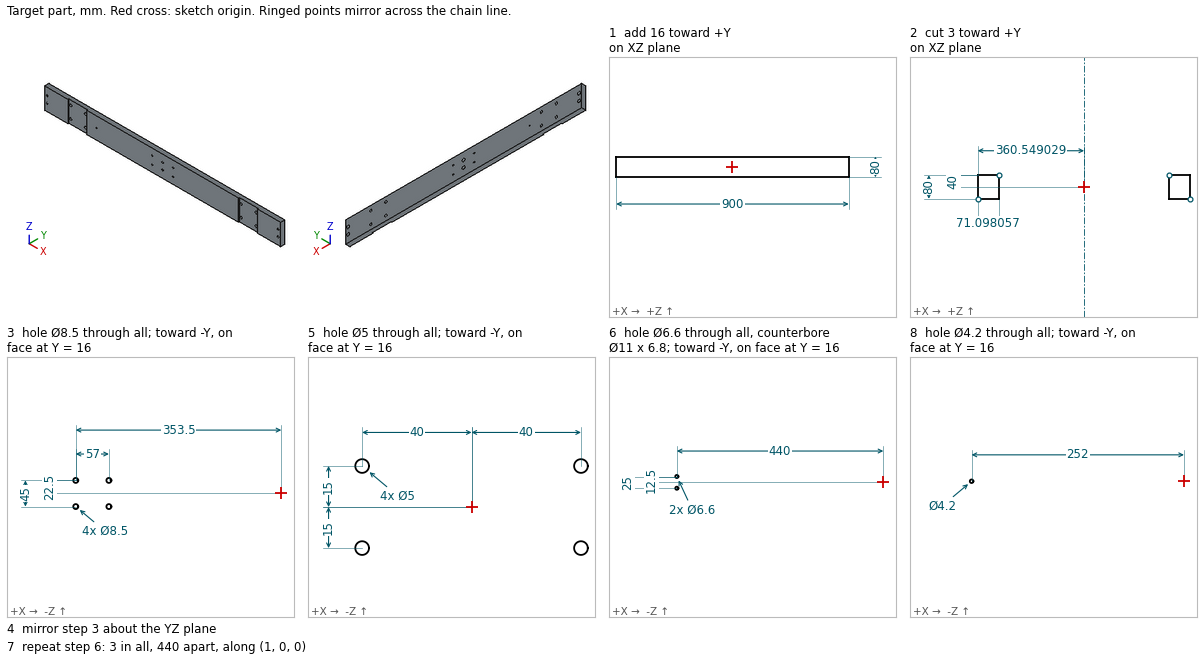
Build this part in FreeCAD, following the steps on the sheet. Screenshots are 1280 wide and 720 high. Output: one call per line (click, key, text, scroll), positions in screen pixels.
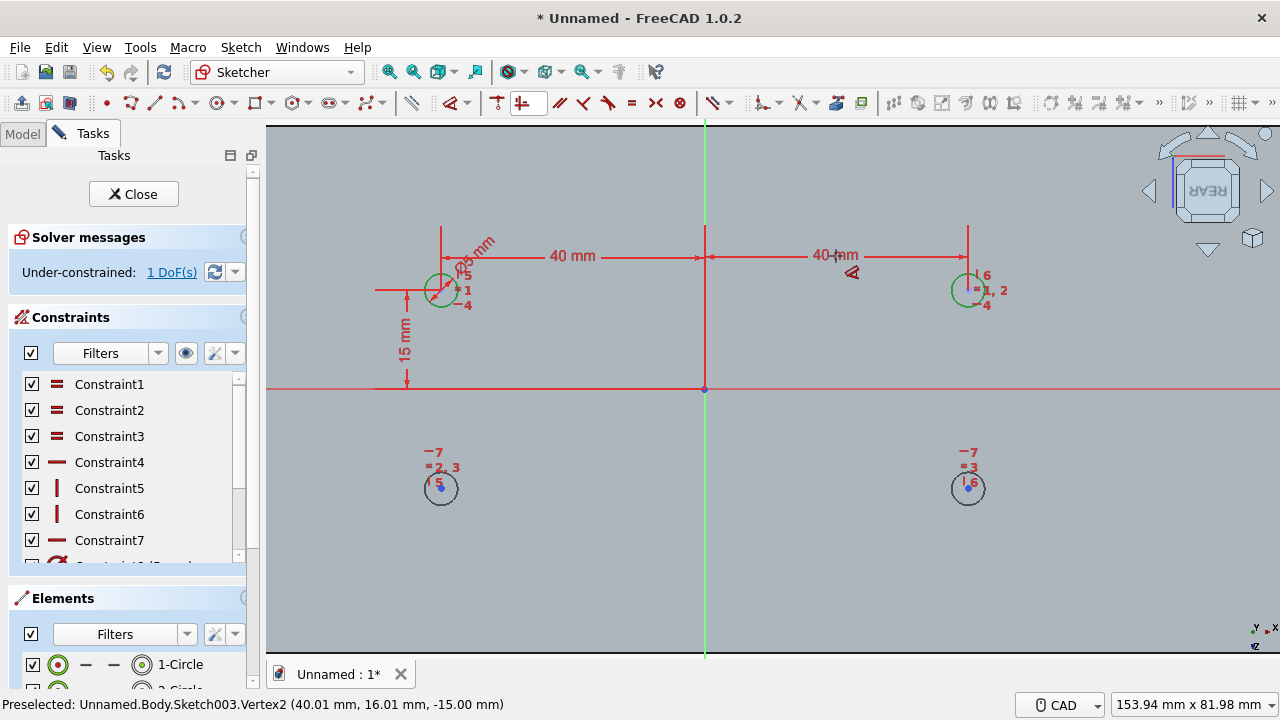
click(441, 489)
click(407, 439)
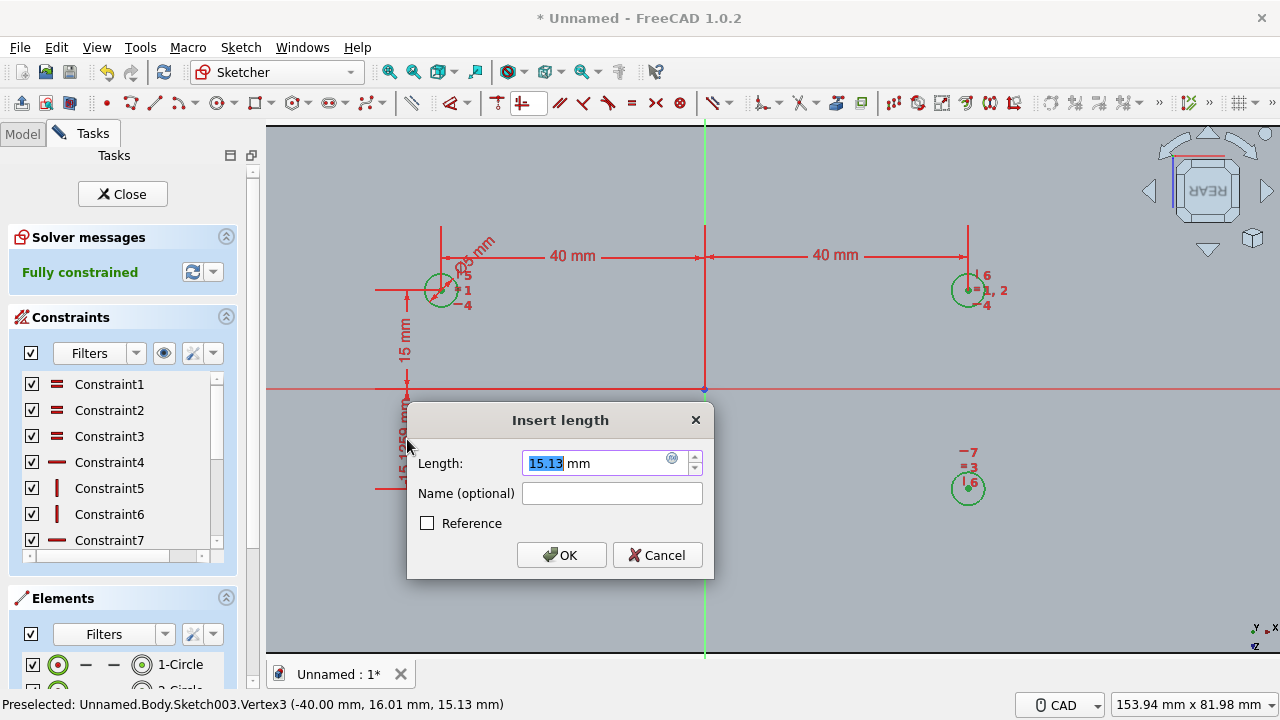
text(15)
key(Return)
key(Escape)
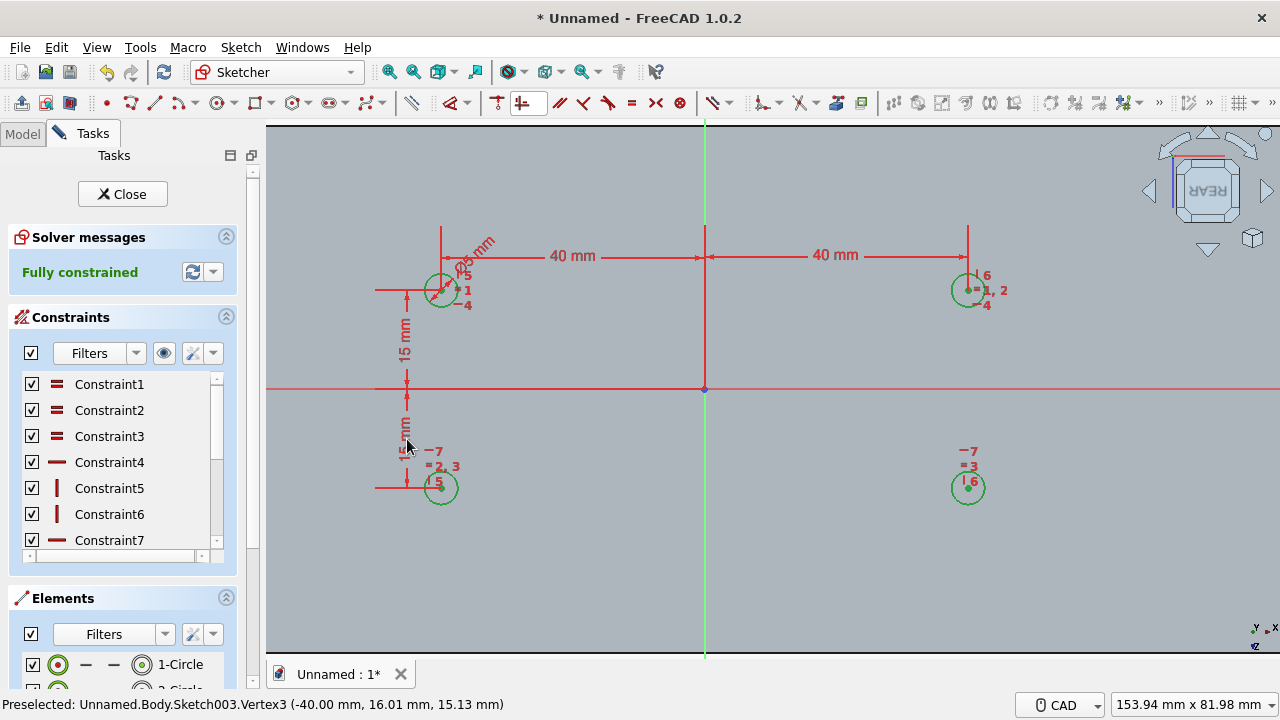
click(123, 194)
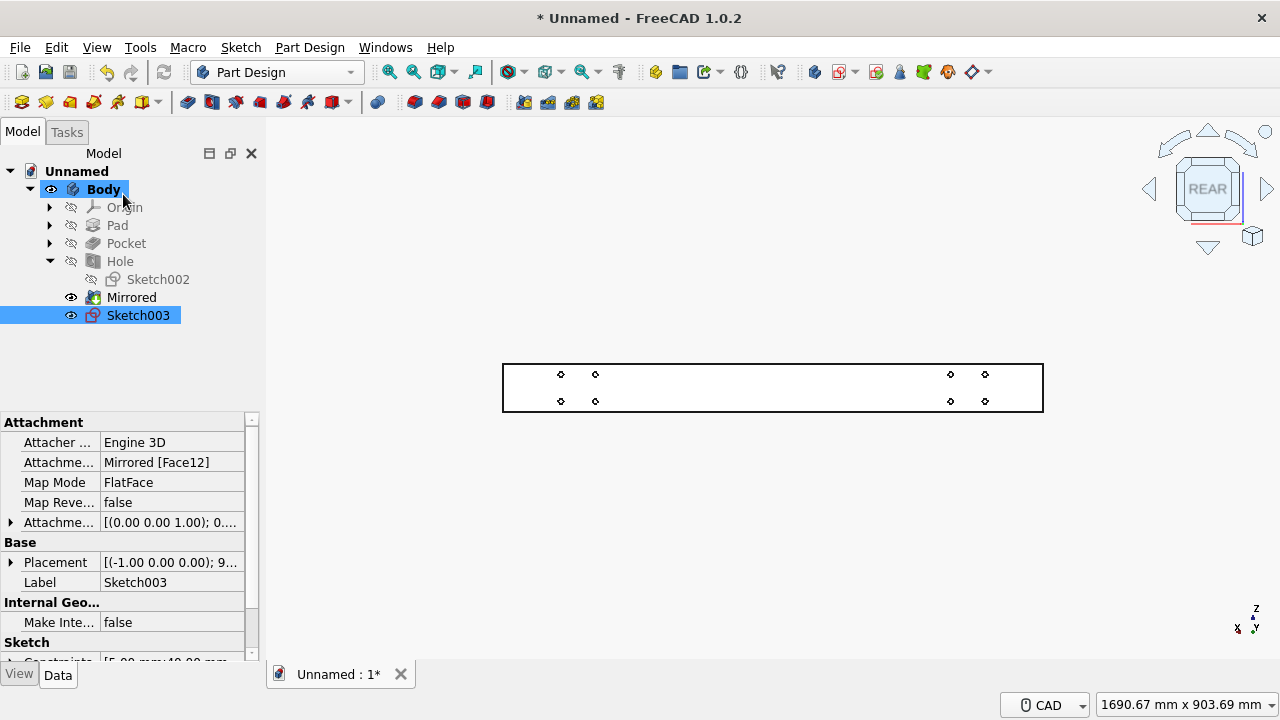
click(212, 102)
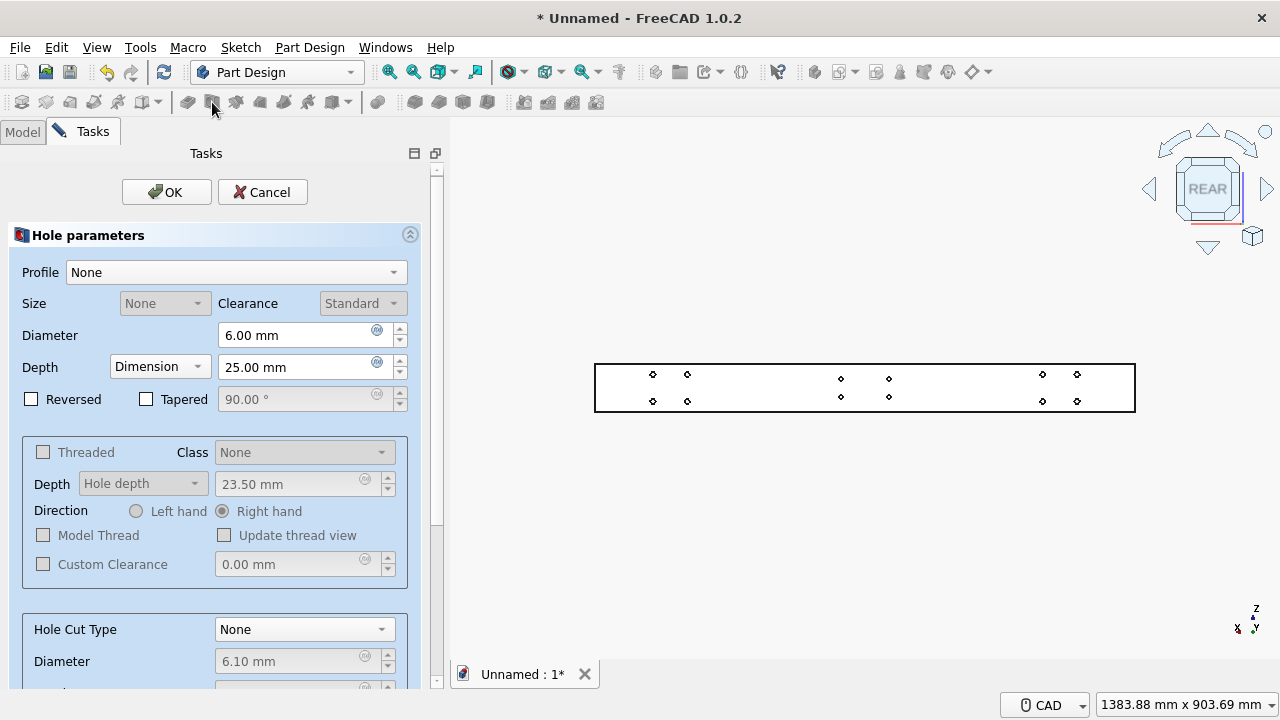
triple_click(305, 335)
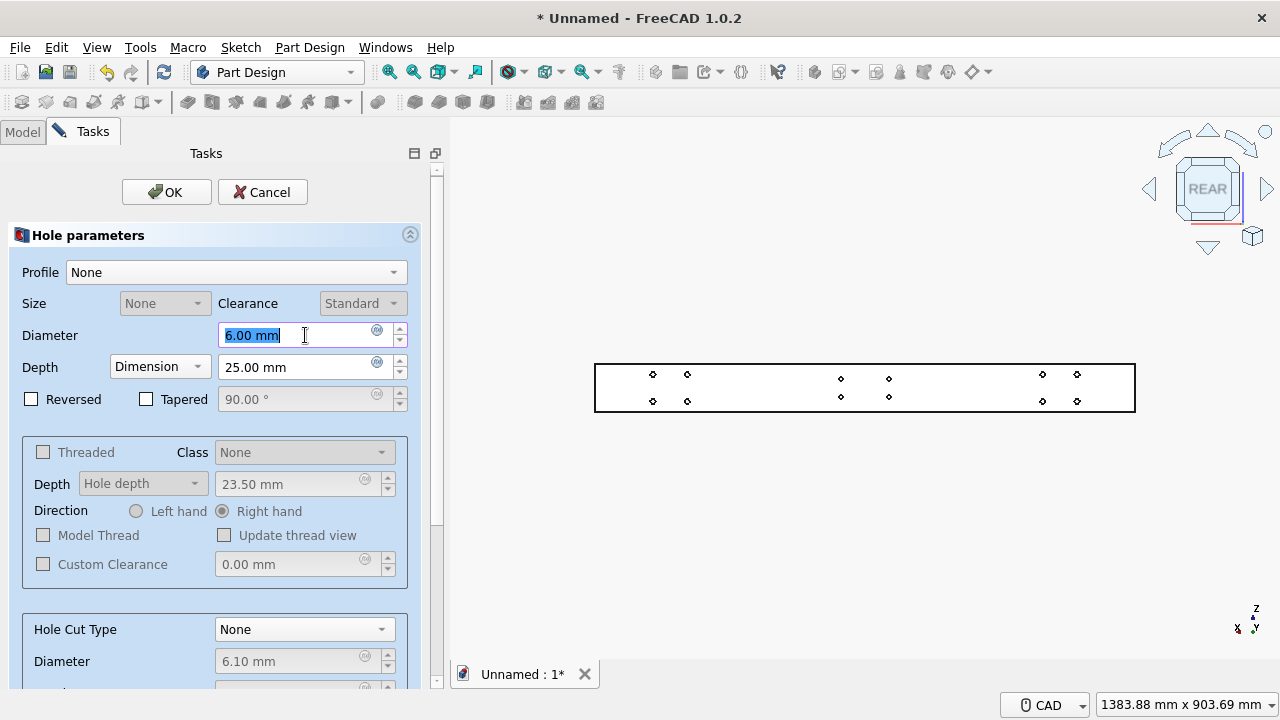
text(5)
key(Tab)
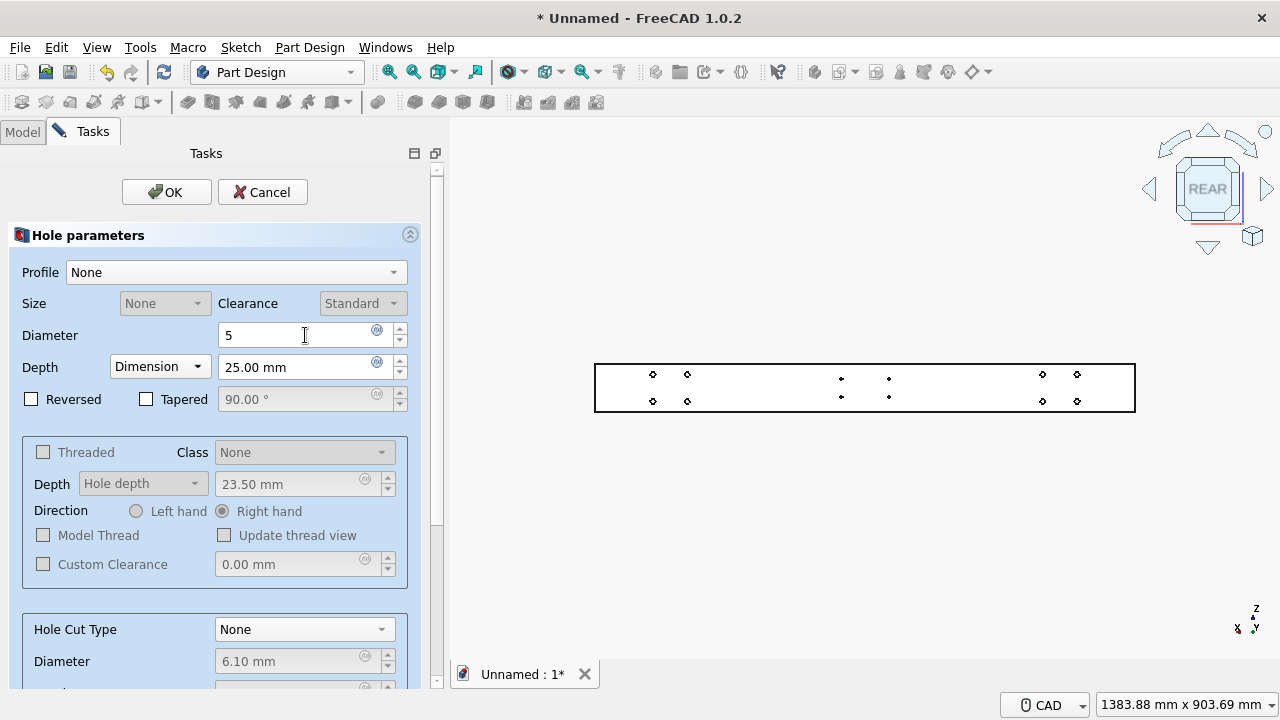
click(161, 366)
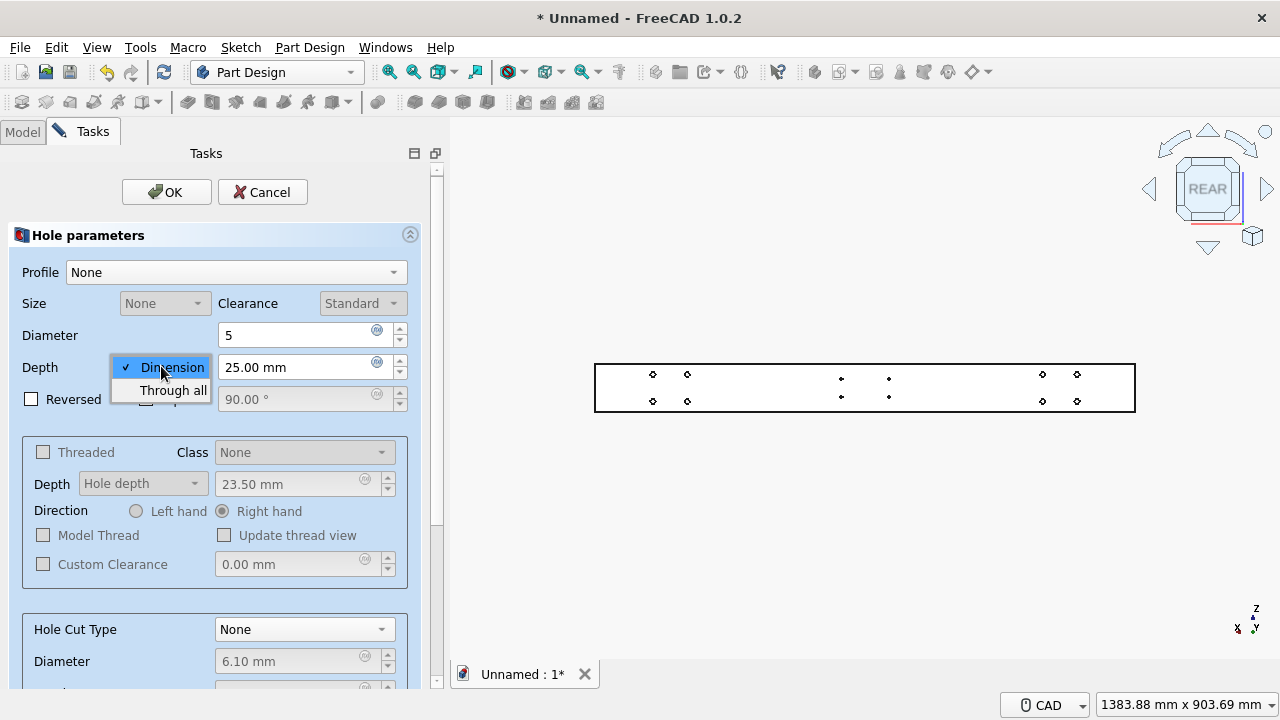
click(160, 390)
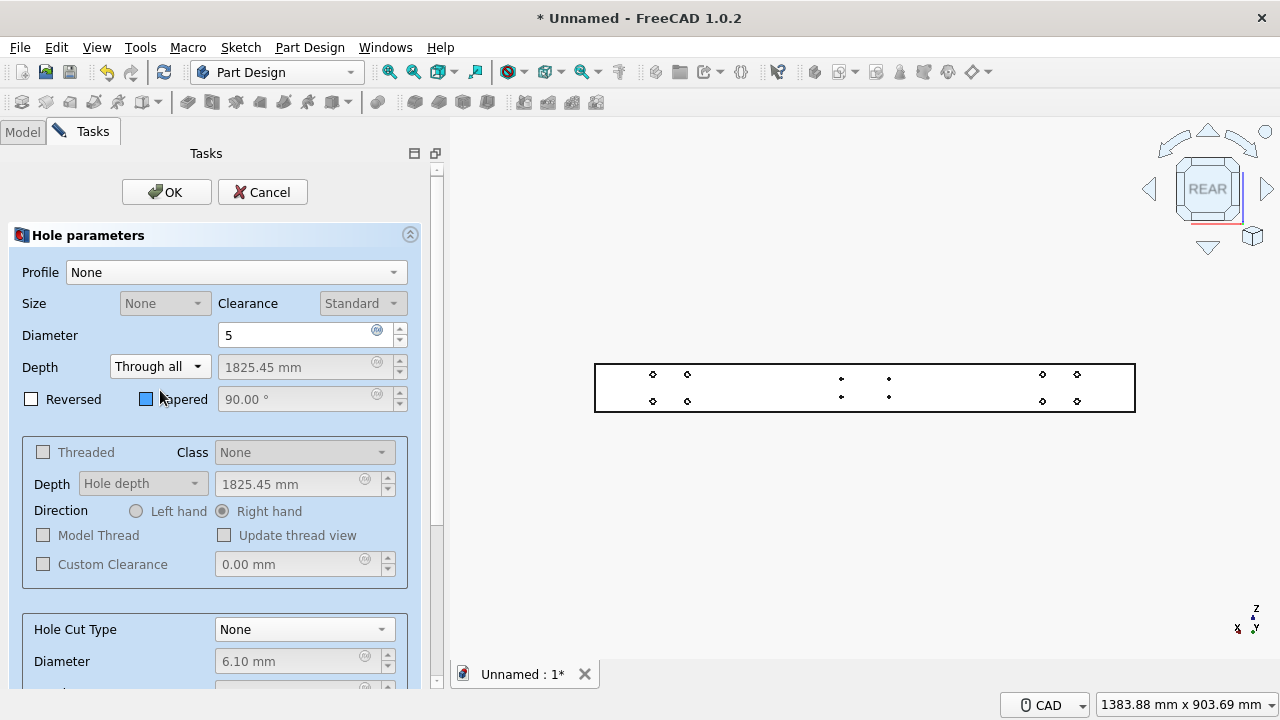
click(167, 192)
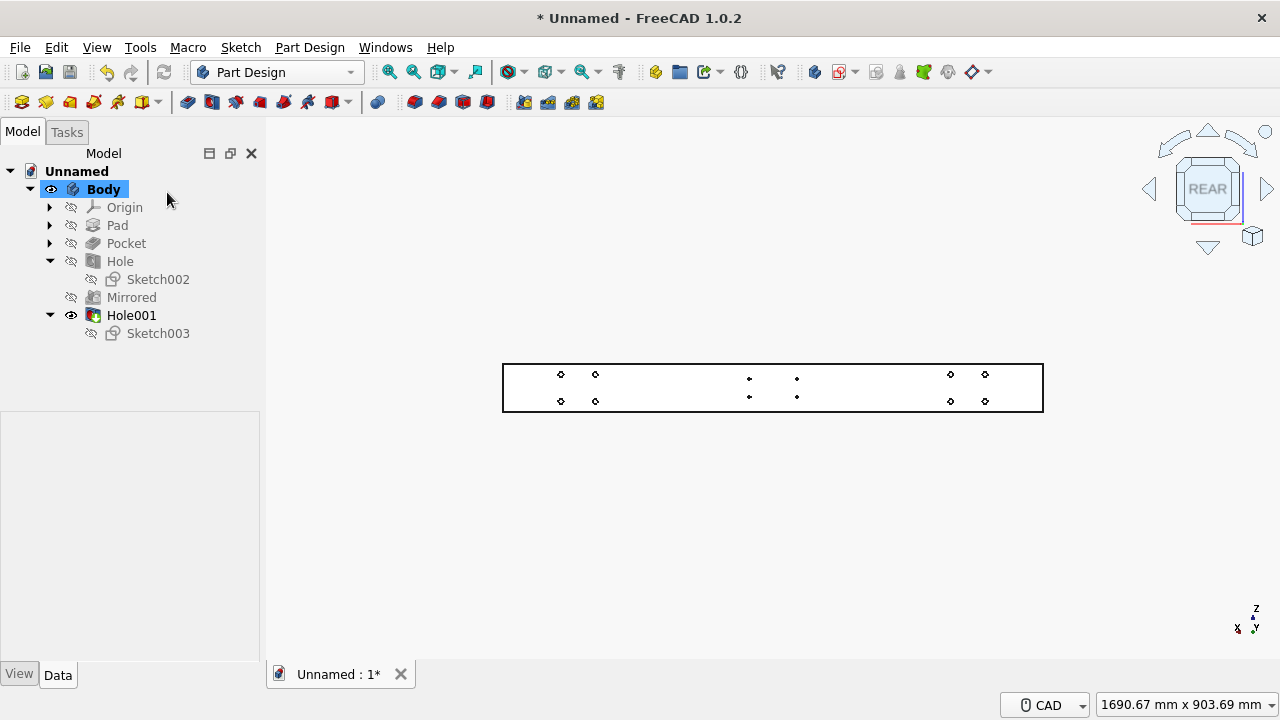
click(619, 387)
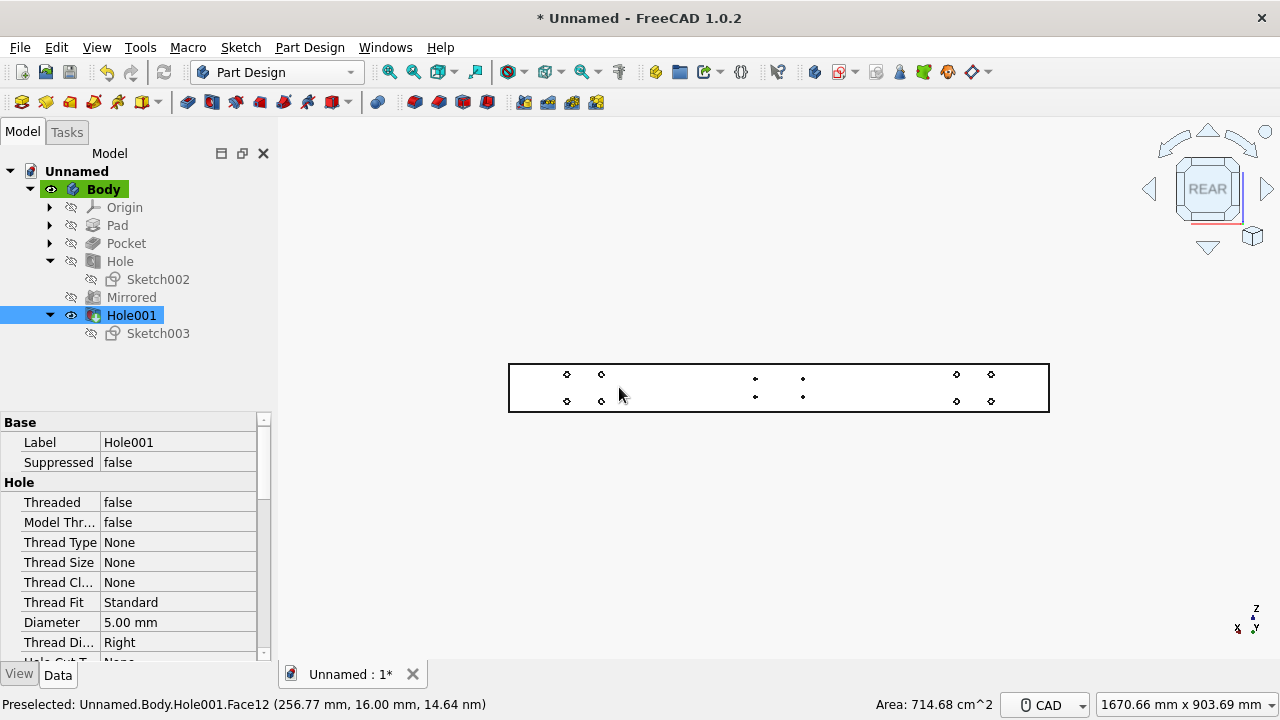
click(840, 72)